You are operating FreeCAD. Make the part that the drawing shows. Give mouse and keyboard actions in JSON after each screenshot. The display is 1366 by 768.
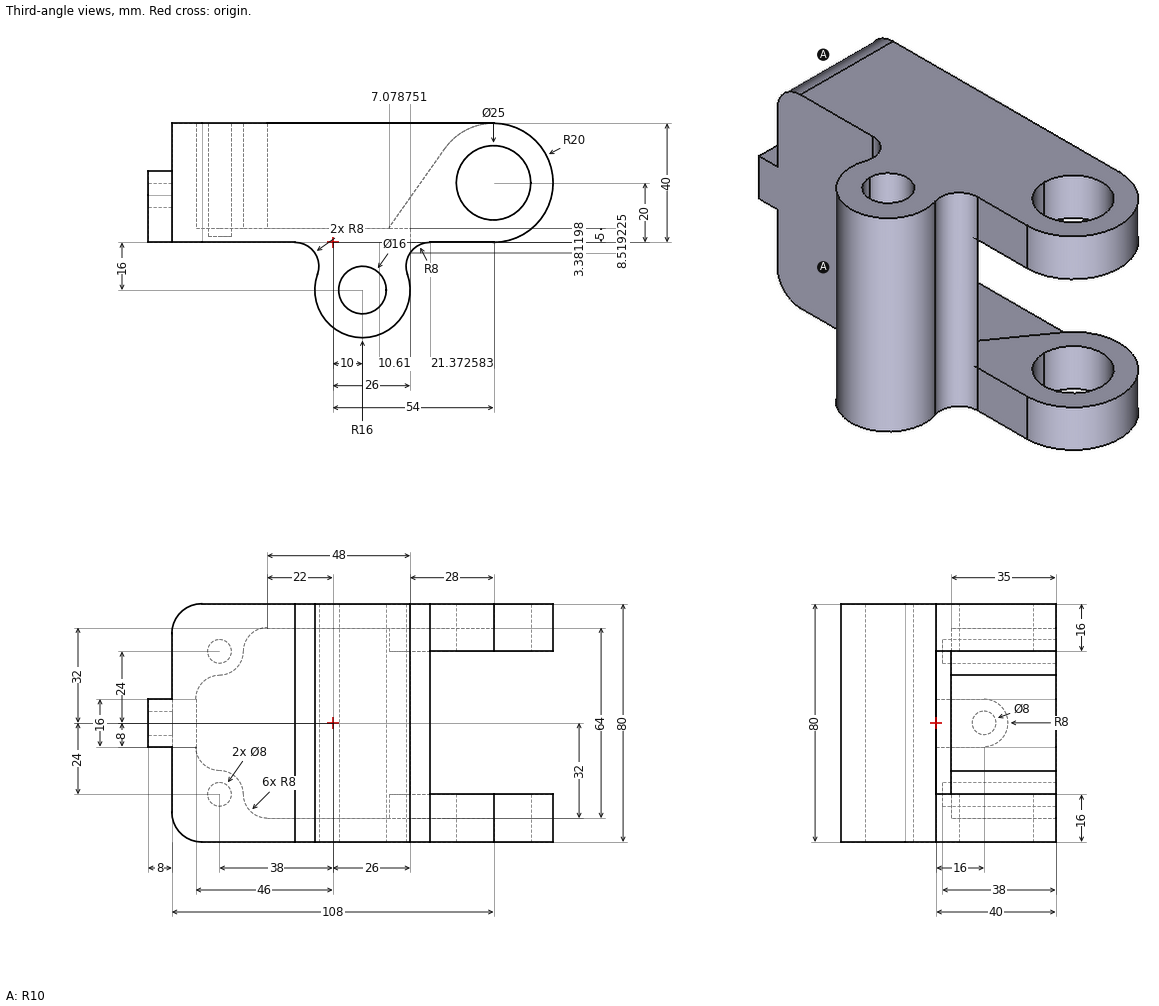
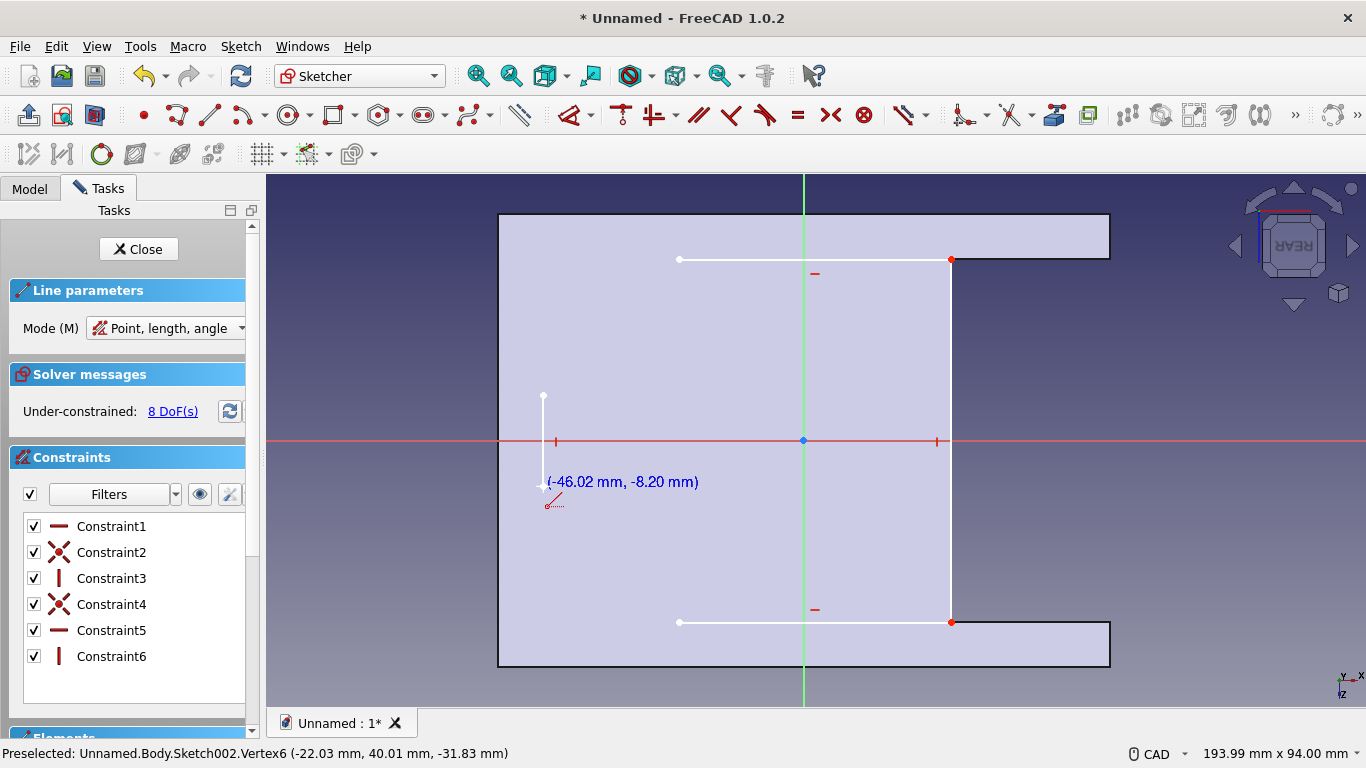
{"action": "key", "text": "g 3 a"}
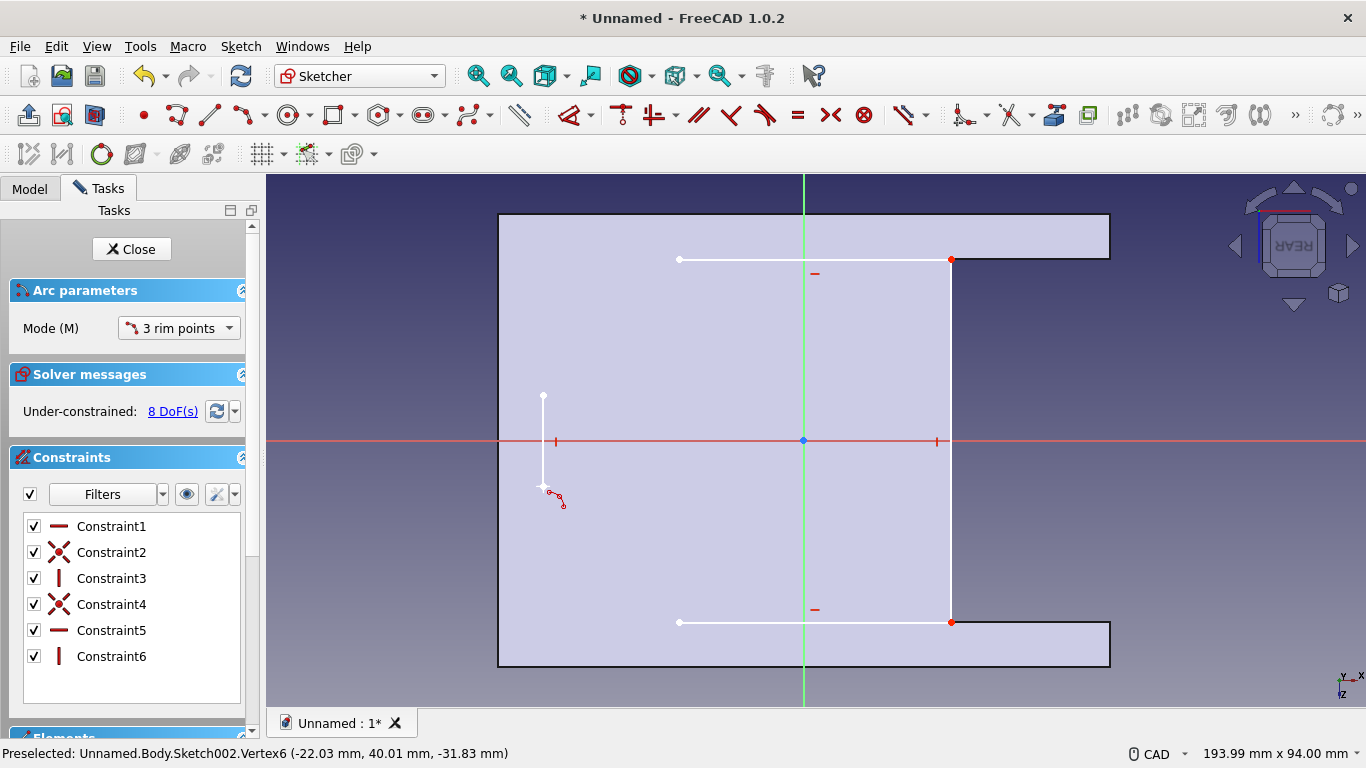
{"action": "left_click", "coordinate": [679, 260]}
{"action": "left_click", "coordinate": [634, 304]}
{"action": "left_click", "coordinate": [647, 272]}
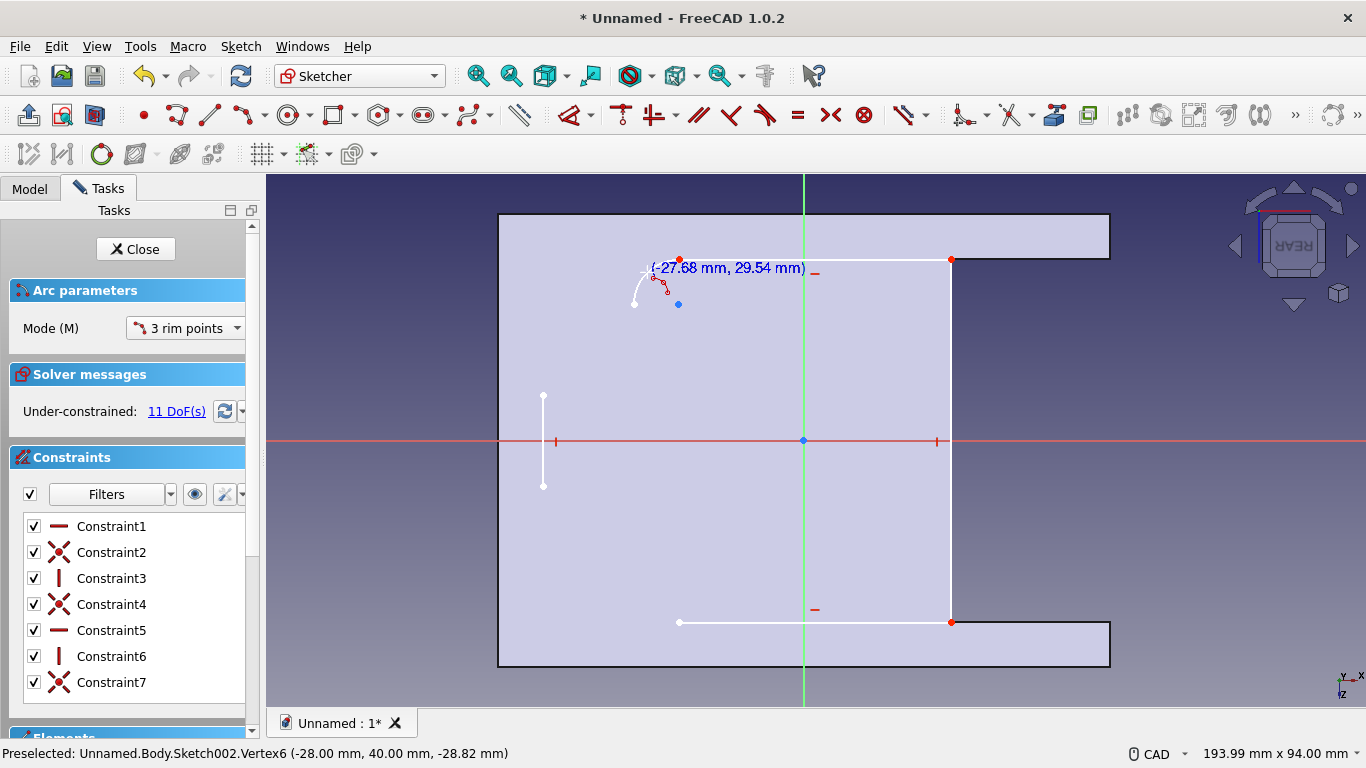
{"action": "left_click", "coordinate": [634, 305]}
{"action": "left_click", "coordinate": [588, 350]}
{"action": "left_click", "coordinate": [621, 336]}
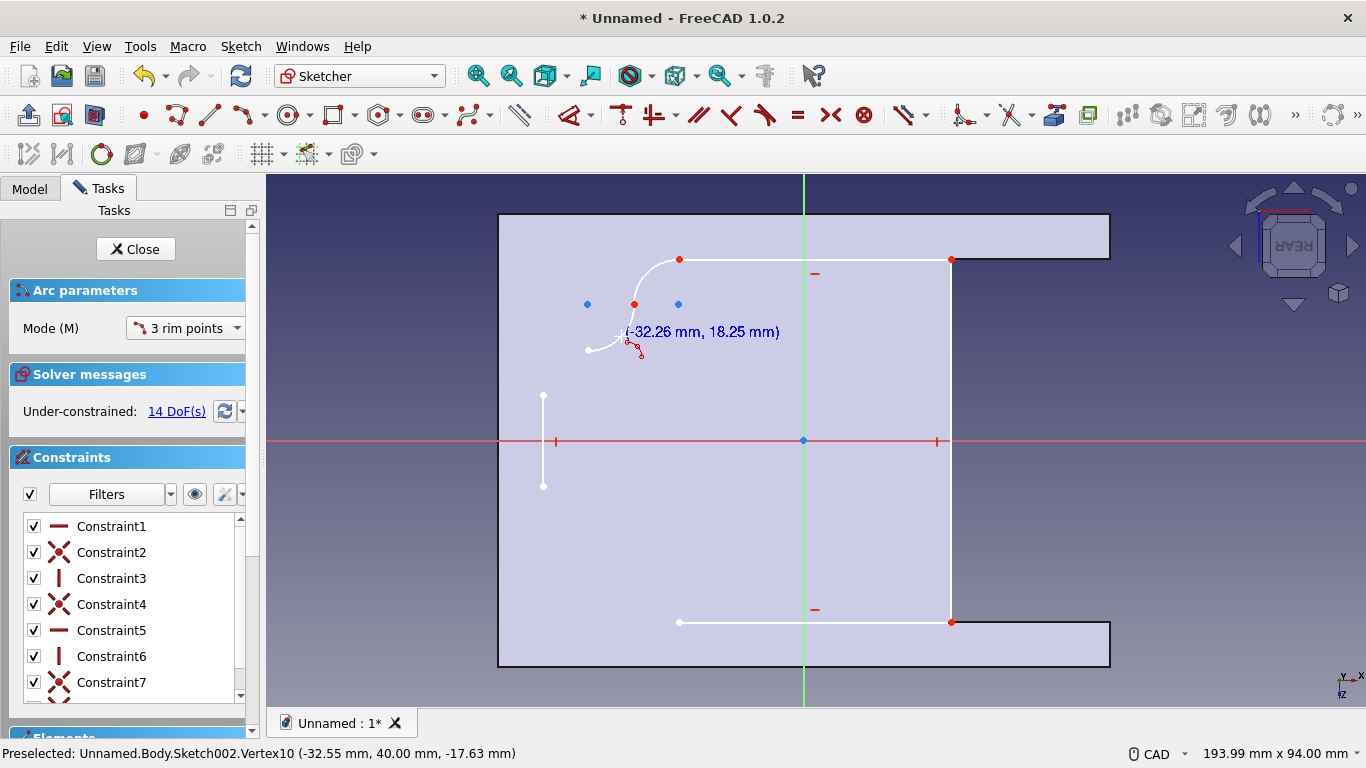
{"action": "left_click", "coordinate": [588, 351]}
{"action": "left_click", "coordinate": [543, 396]}
{"action": "left_click", "coordinate": [556, 363]}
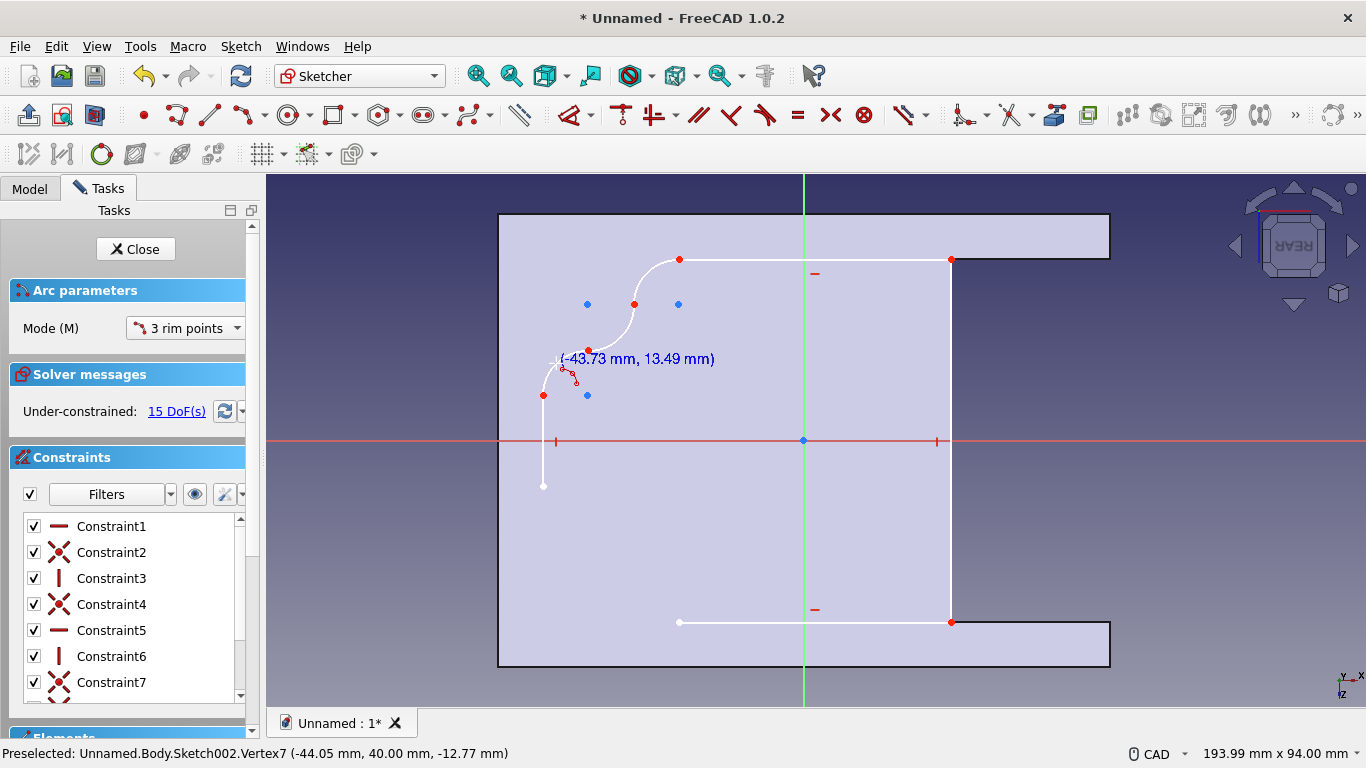
{"action": "left_click", "coordinate": [543, 487]}
{"action": "left_click", "coordinate": [588, 531]}
{"action": "left_click", "coordinate": [556, 518]}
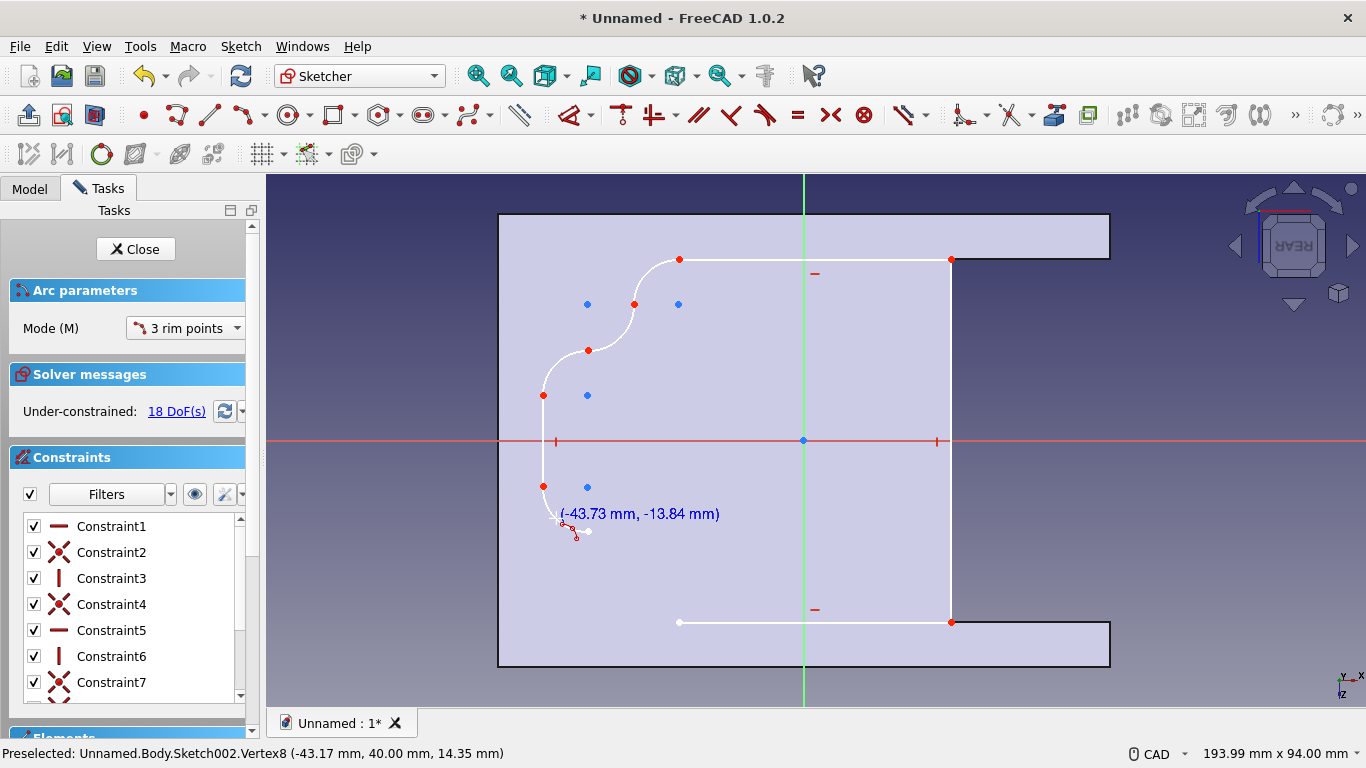
{"action": "left_click", "coordinate": [588, 532]}
{"action": "left_click", "coordinate": [634, 577]}
{"action": "left_click", "coordinate": [621, 545]}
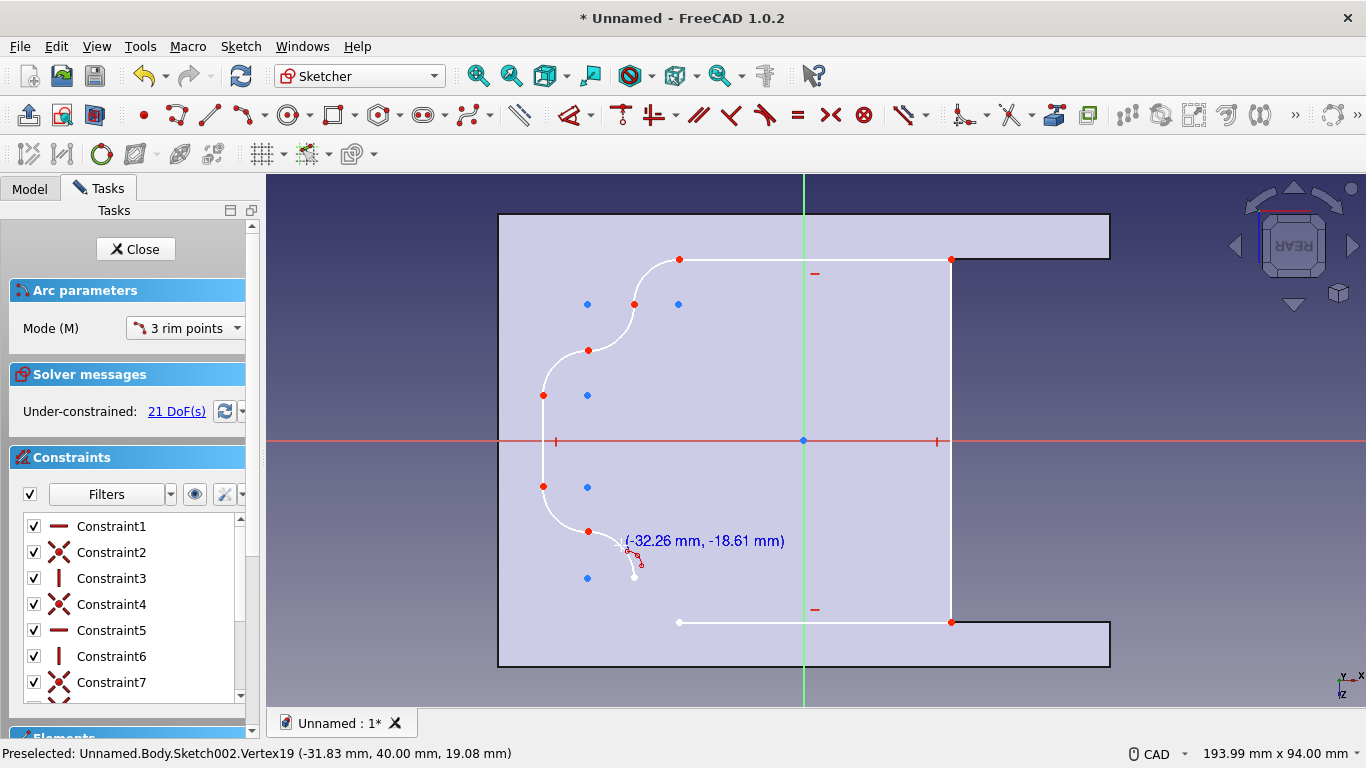
{"action": "left_click", "coordinate": [634, 578]}
{"action": "left_click", "coordinate": [679, 623]}
{"action": "left_click", "coordinate": [647, 609]}
{"action": "key", "text": "Escape"}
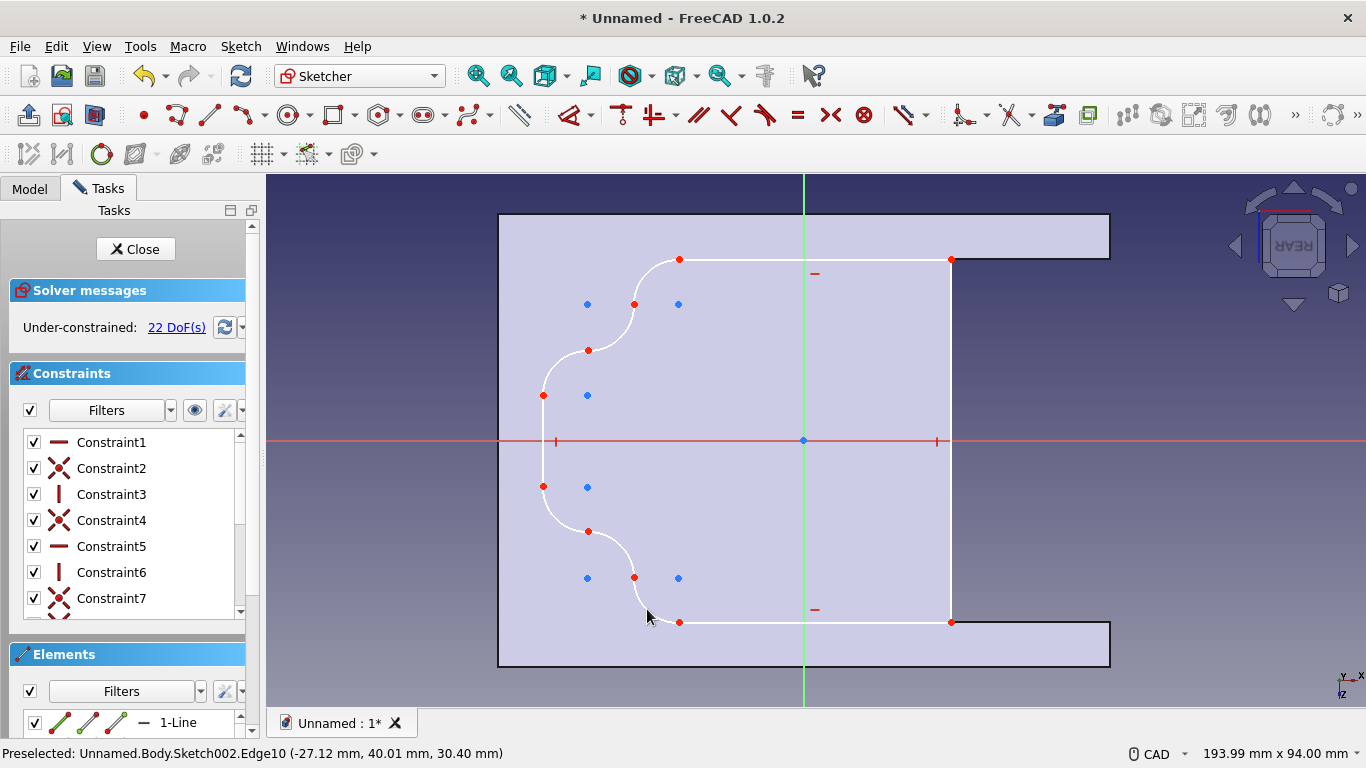
{"action": "left_click", "coordinate": [761, 623]}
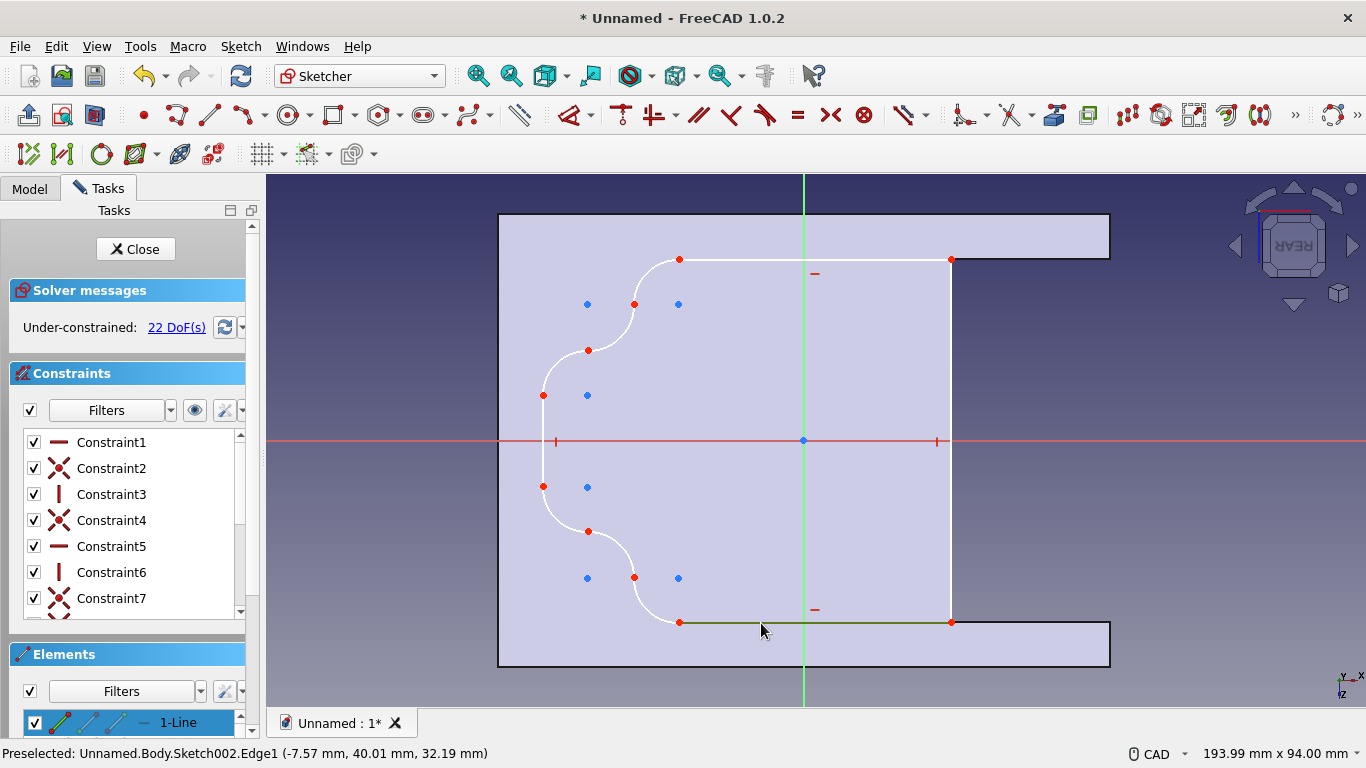
{"action": "left_click", "coordinate": [639, 599]}